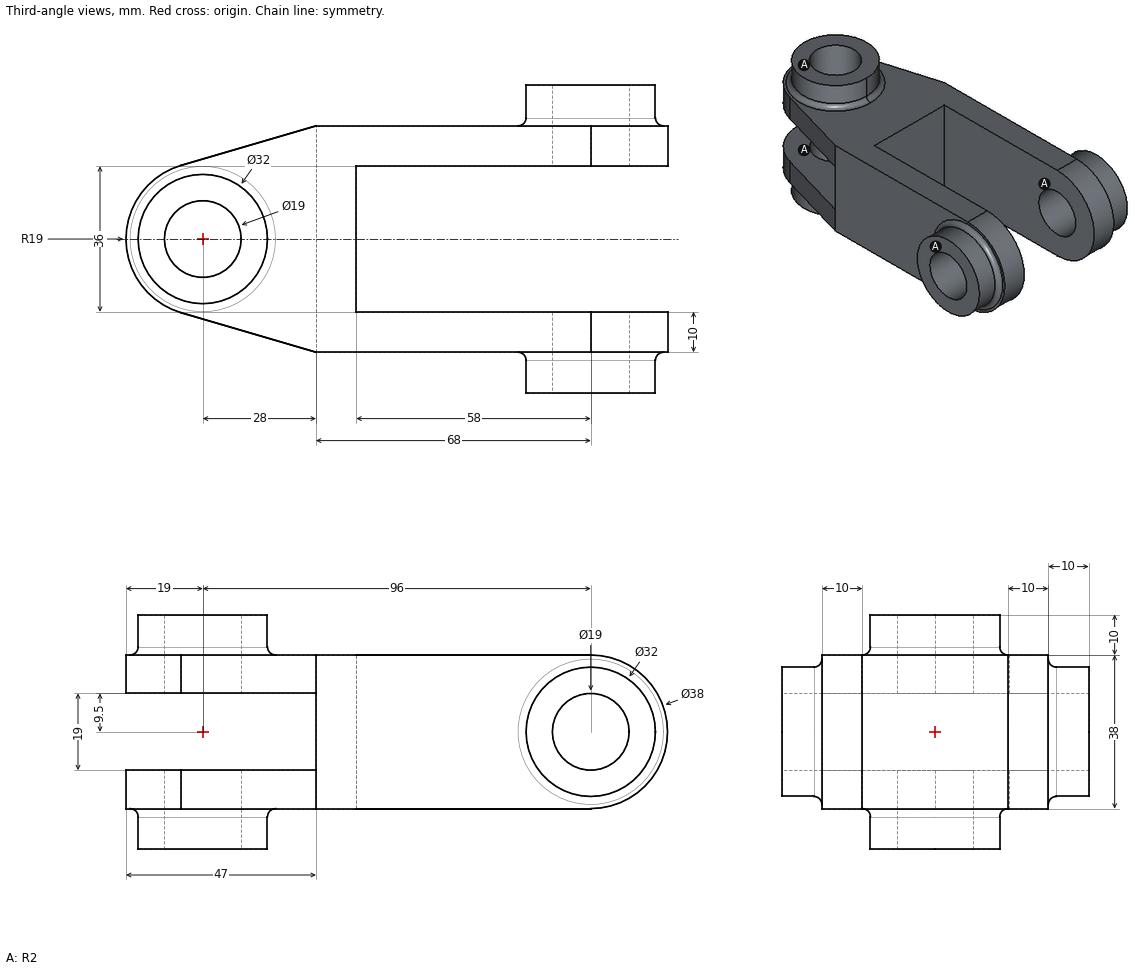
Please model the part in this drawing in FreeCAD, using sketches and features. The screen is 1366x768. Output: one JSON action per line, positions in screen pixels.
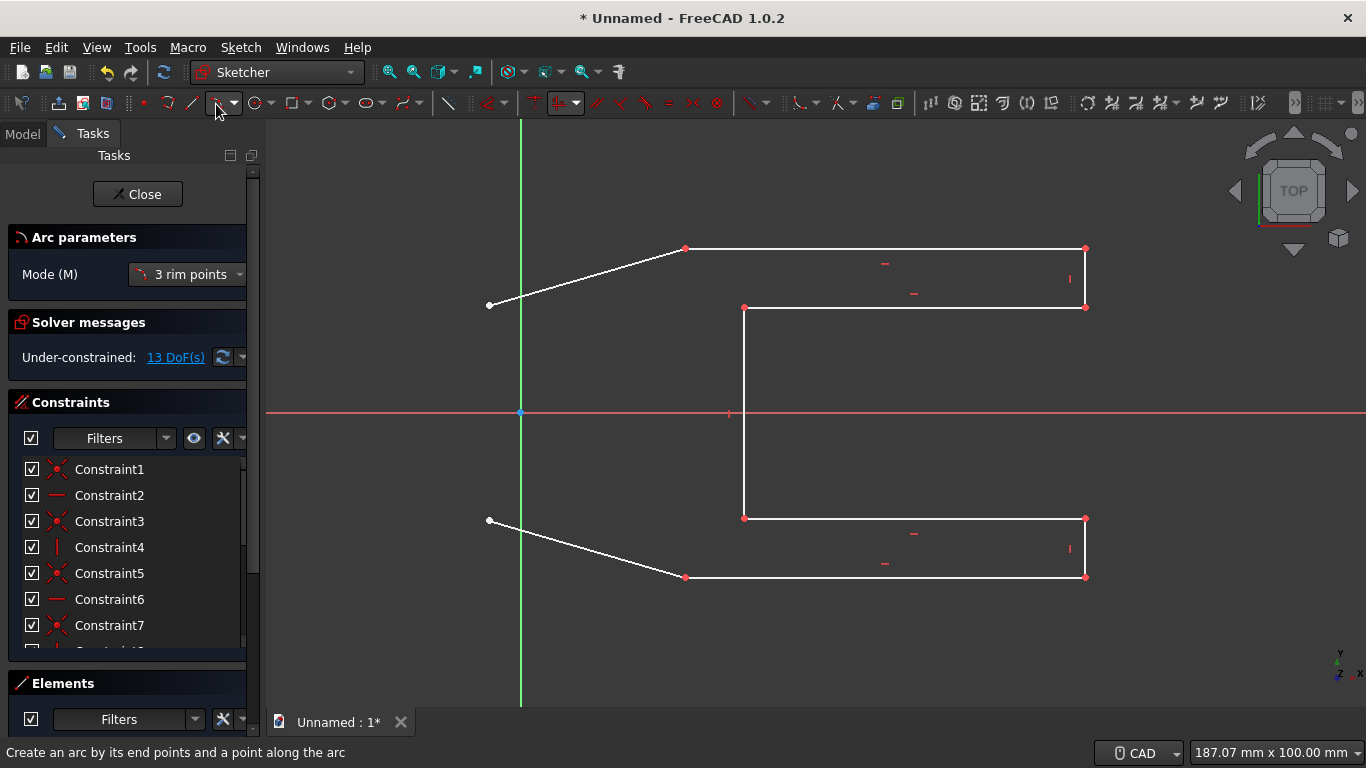
{"action": "left_click", "coordinate": [489, 306]}
{"action": "left_click", "coordinate": [489, 521]}
{"action": "left_click", "coordinate": [413, 384]}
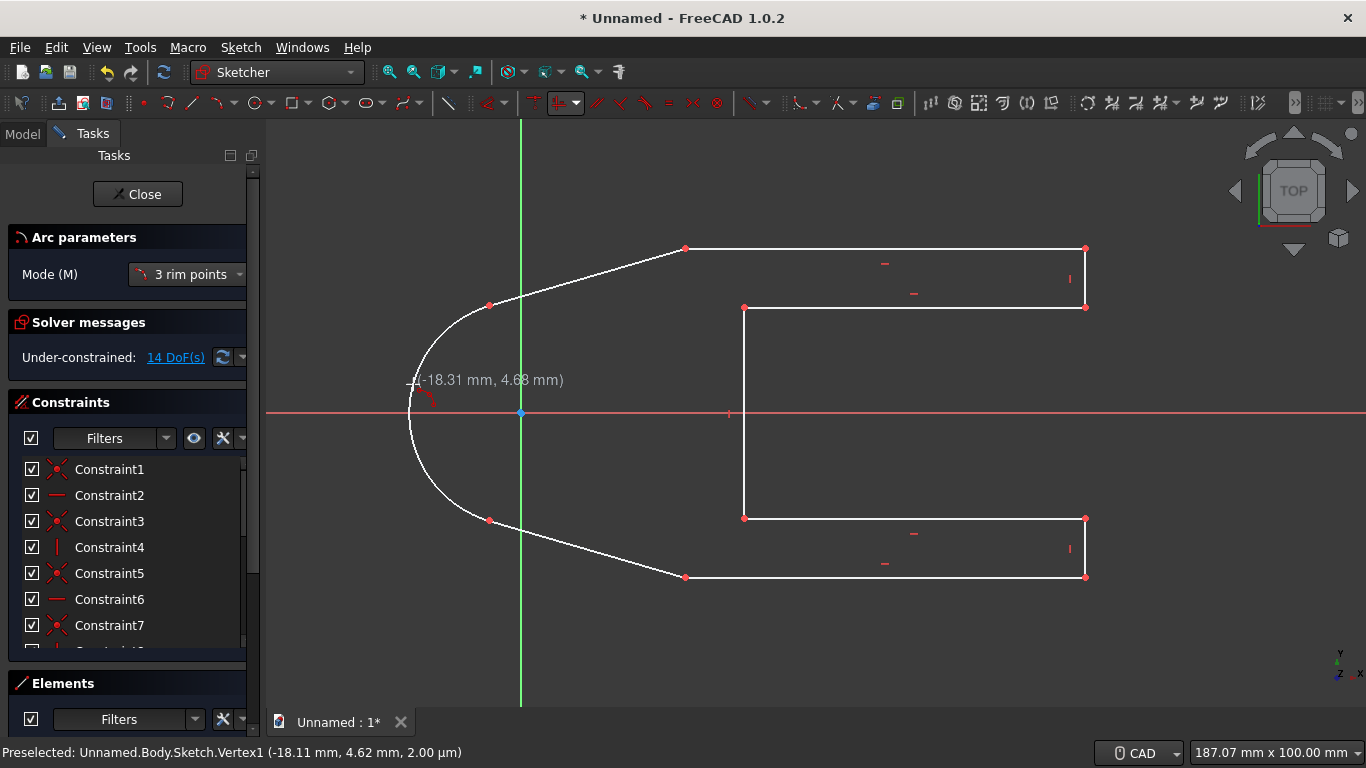
{"action": "key", "text": "g c"}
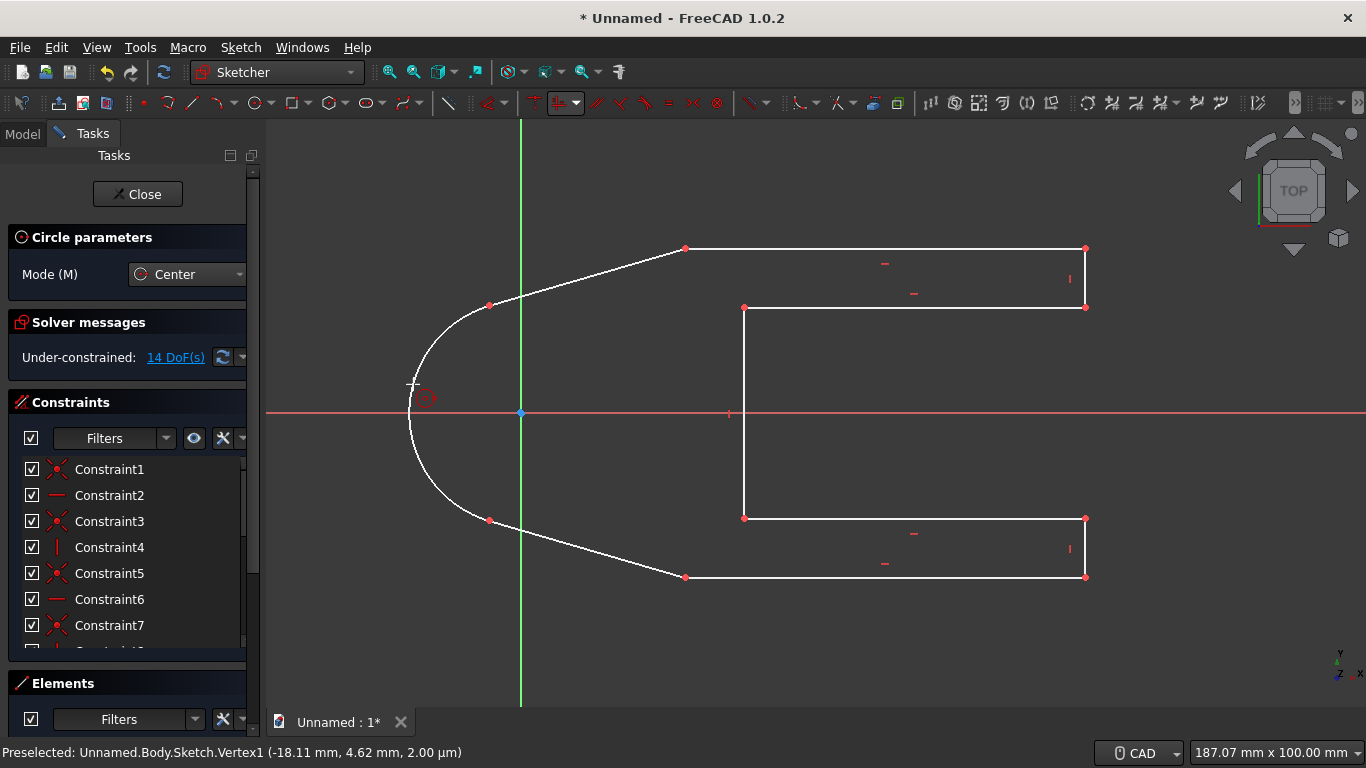
{"action": "left_click", "coordinate": [521, 413]}
{"action": "left_click", "coordinate": [560, 373]}
{"action": "key", "text": "Escape"}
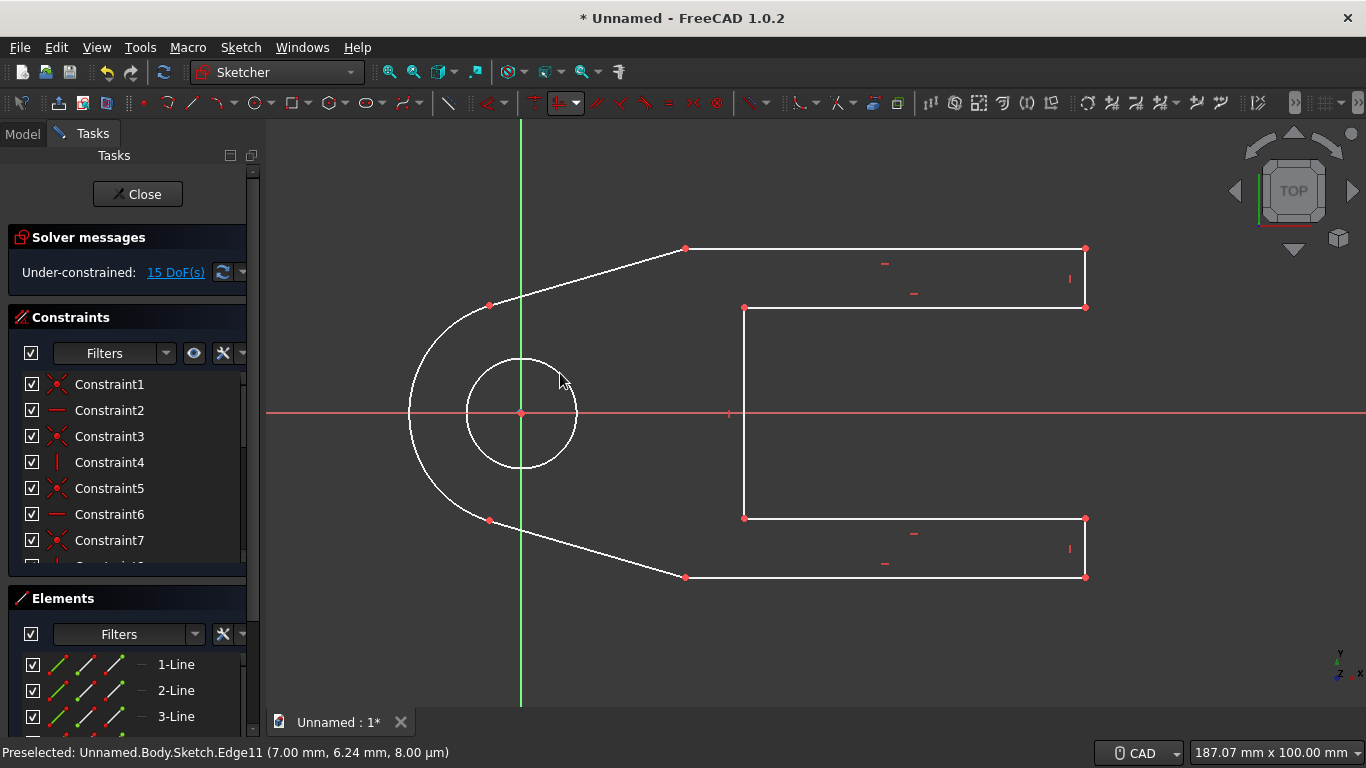
{"action": "left_click", "coordinate": [548, 538]}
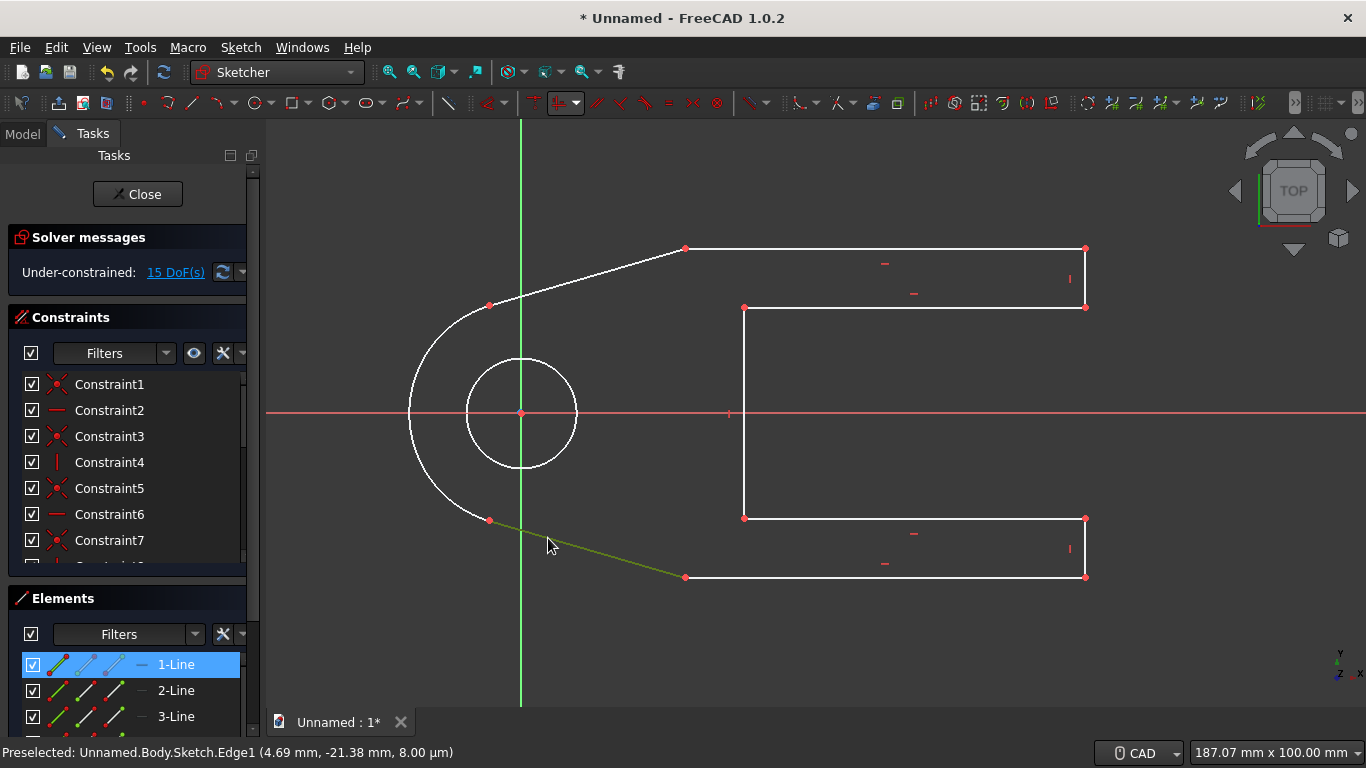
{"action": "left_click", "coordinate": [424, 359]}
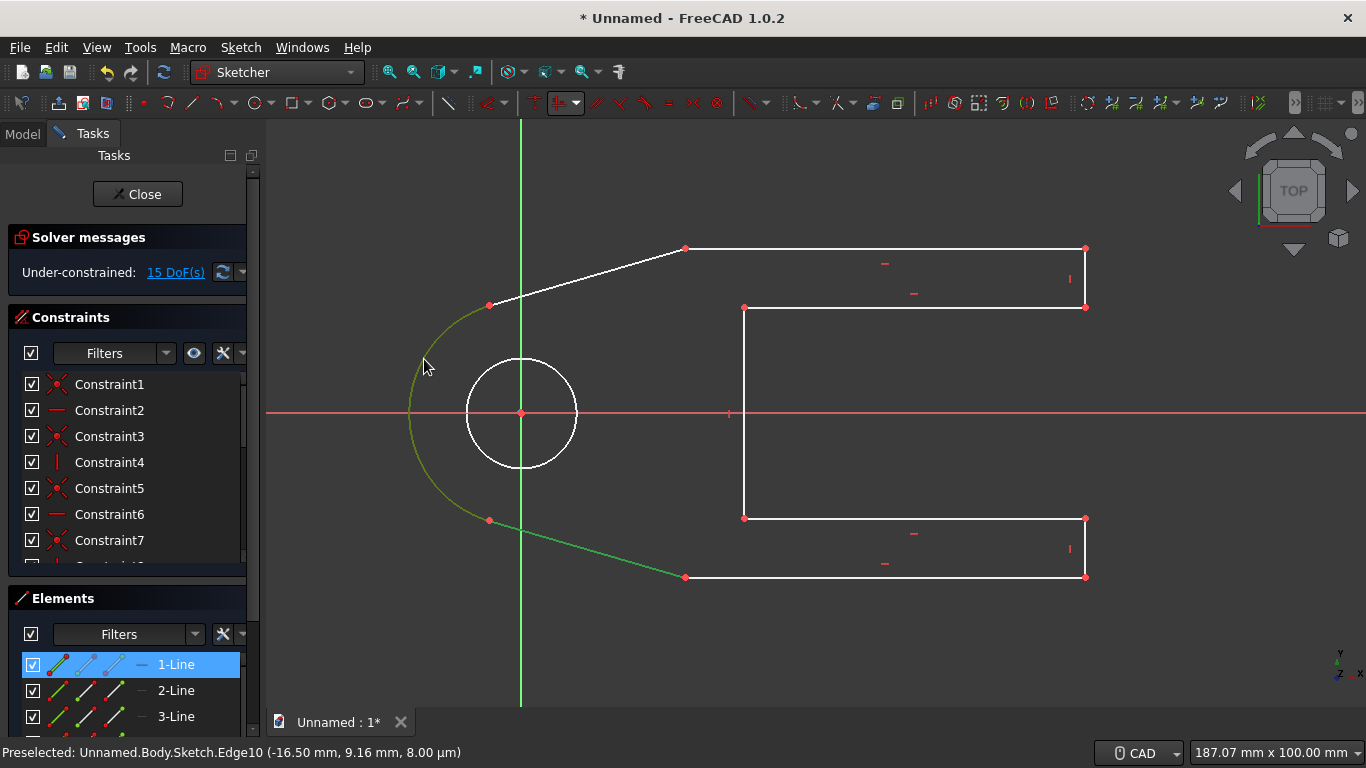
{"action": "left_click", "coordinate": [646, 104]}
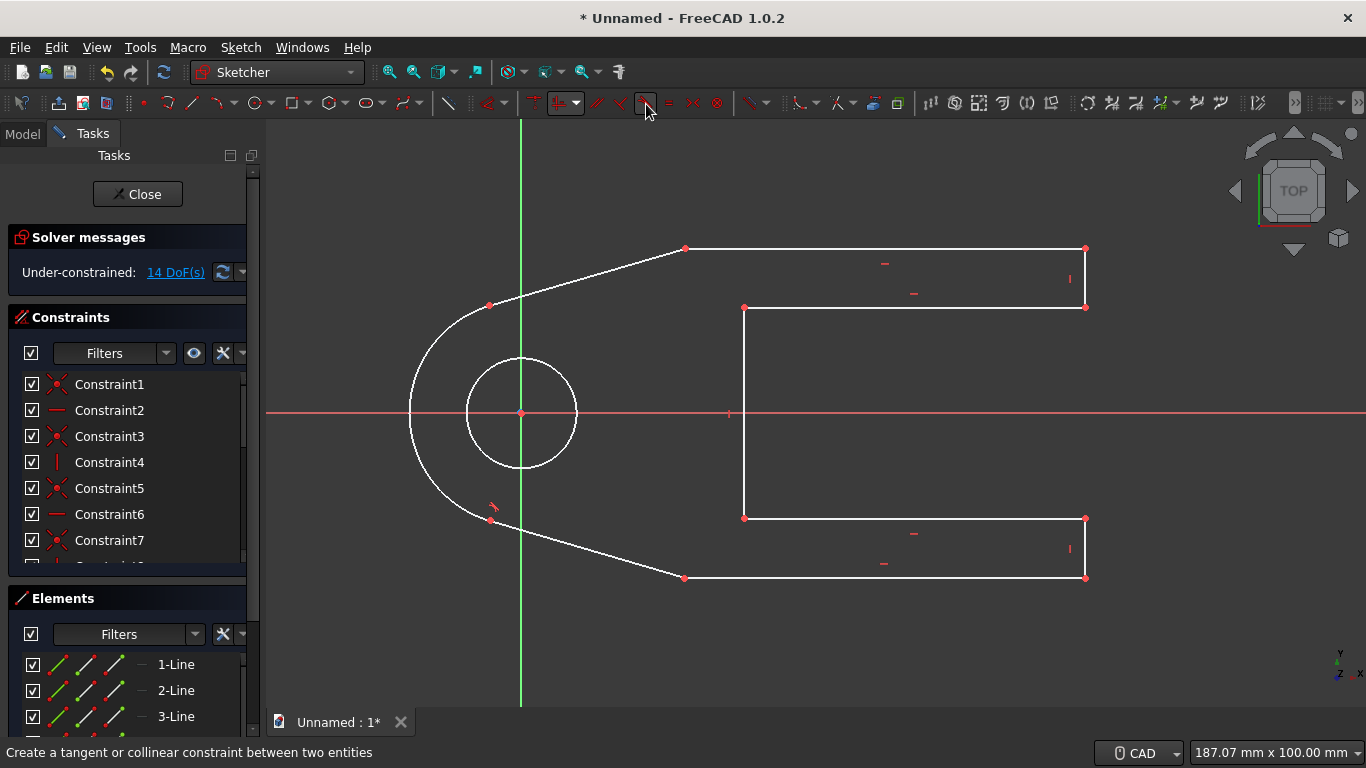
{"action": "left_click", "coordinate": [626, 266]}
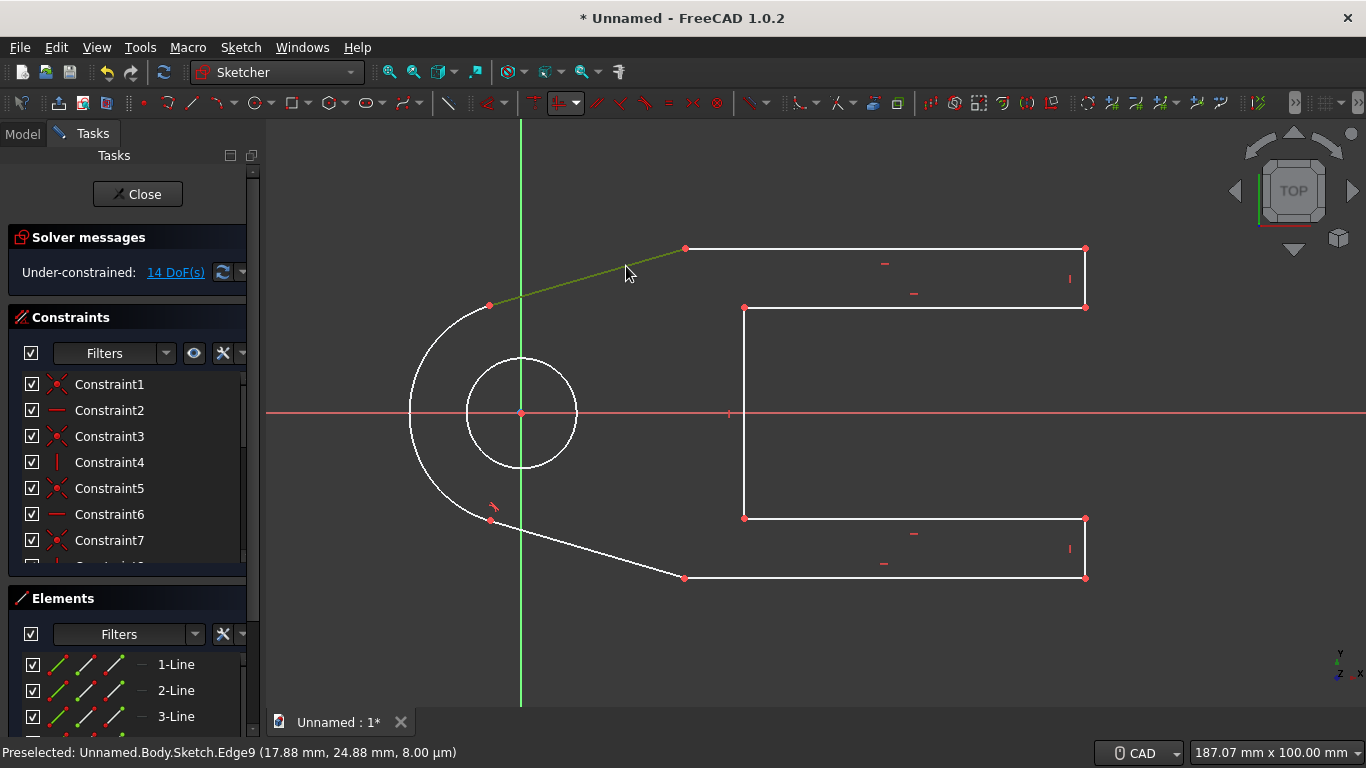
{"action": "left_click", "coordinate": [424, 359]}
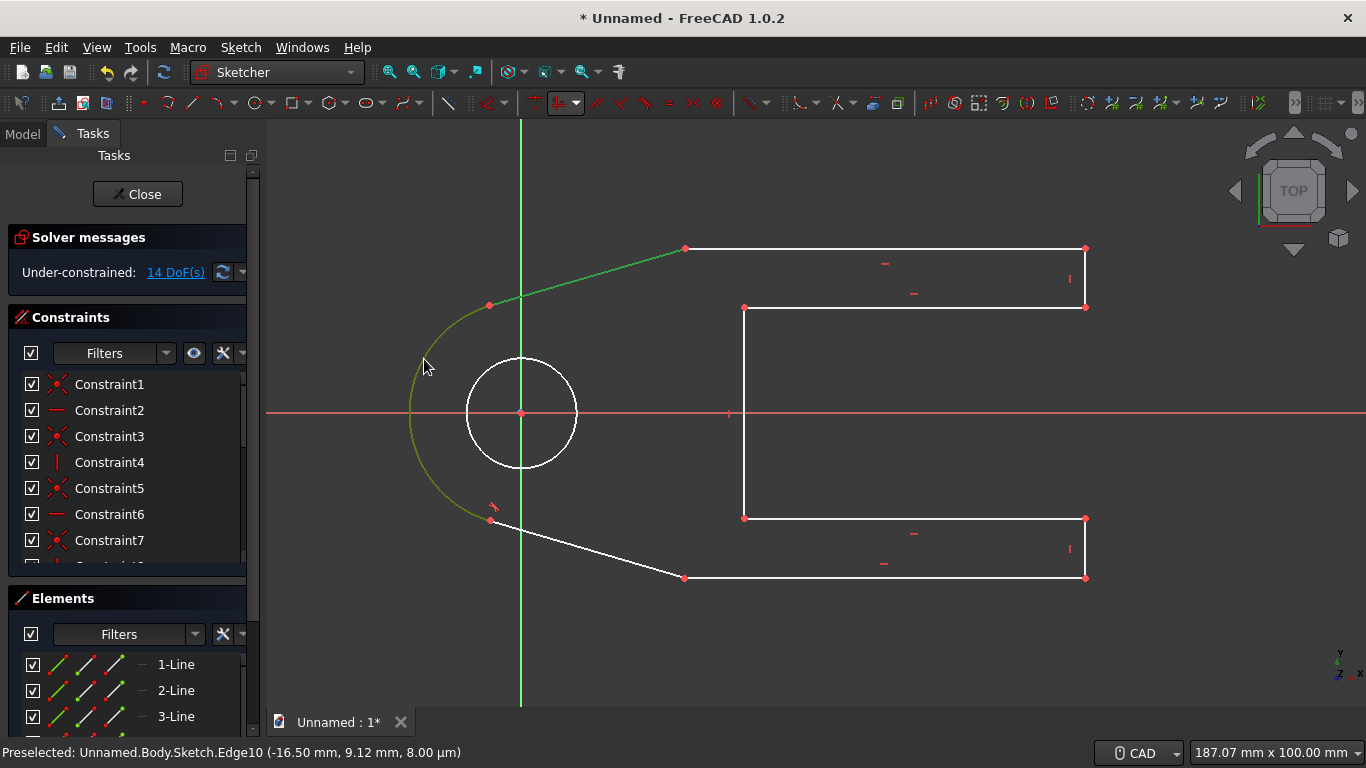
{"action": "left_click", "coordinate": [646, 104]}